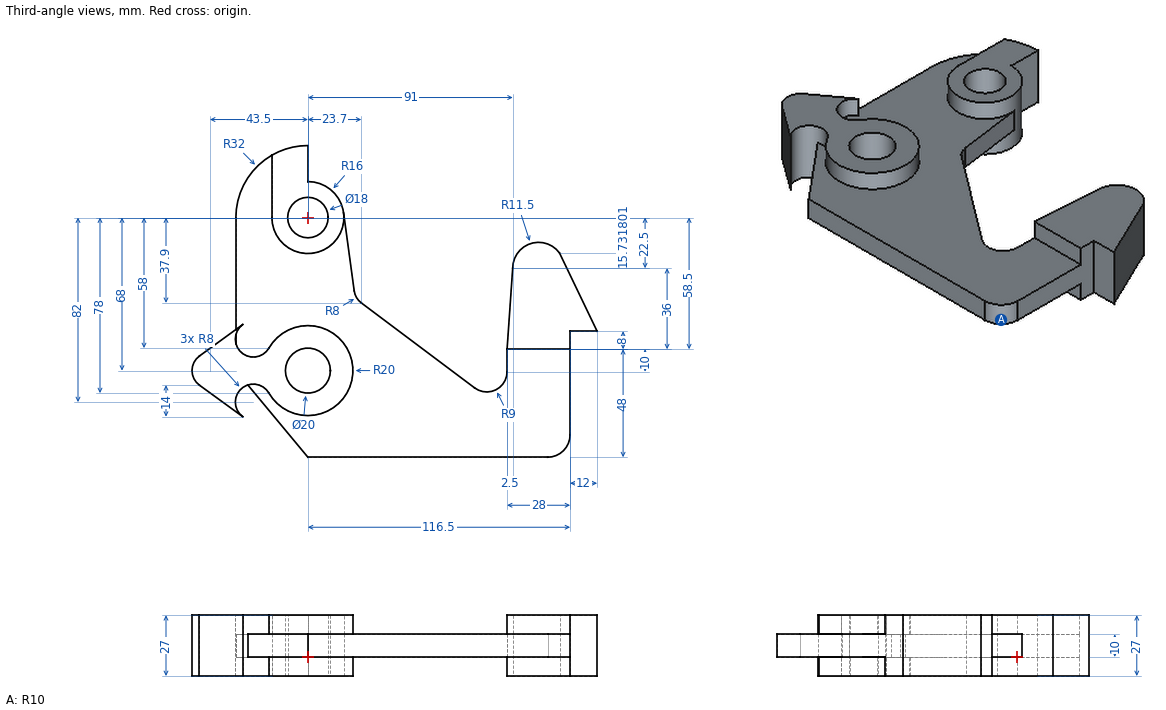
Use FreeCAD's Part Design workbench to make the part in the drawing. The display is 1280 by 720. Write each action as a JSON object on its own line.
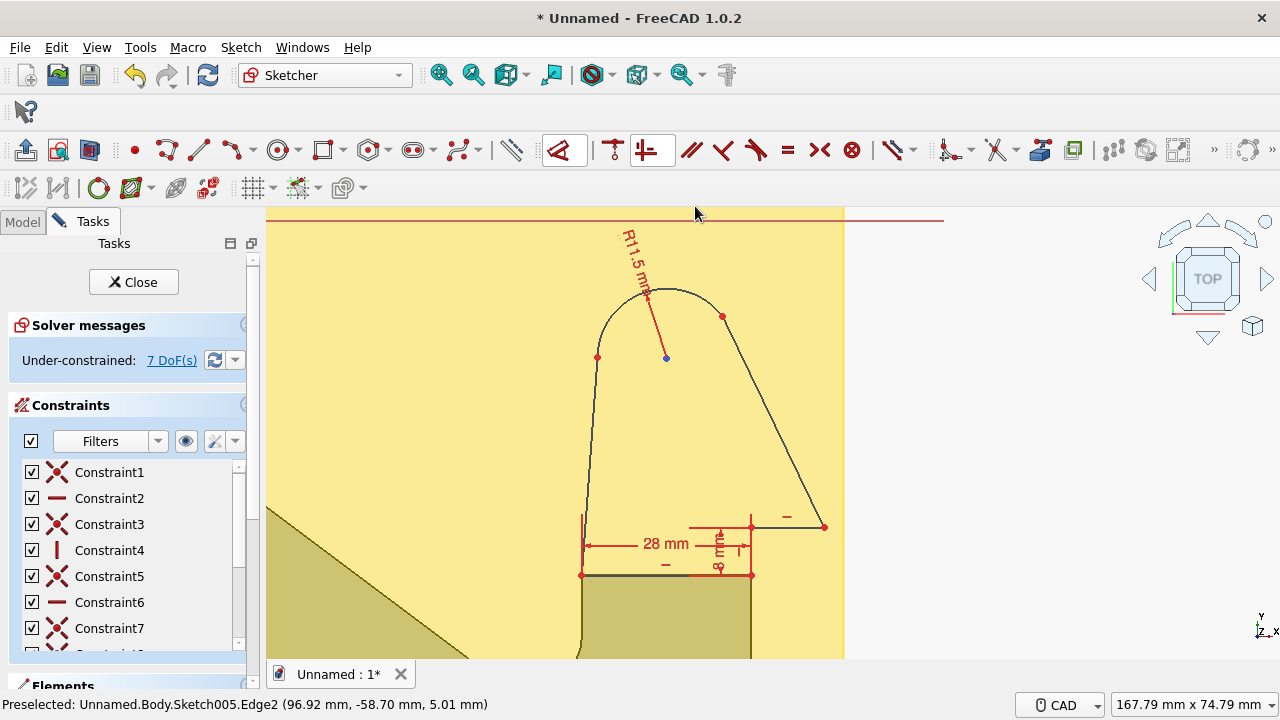
{"action": "left_click", "coordinate": [773, 528]}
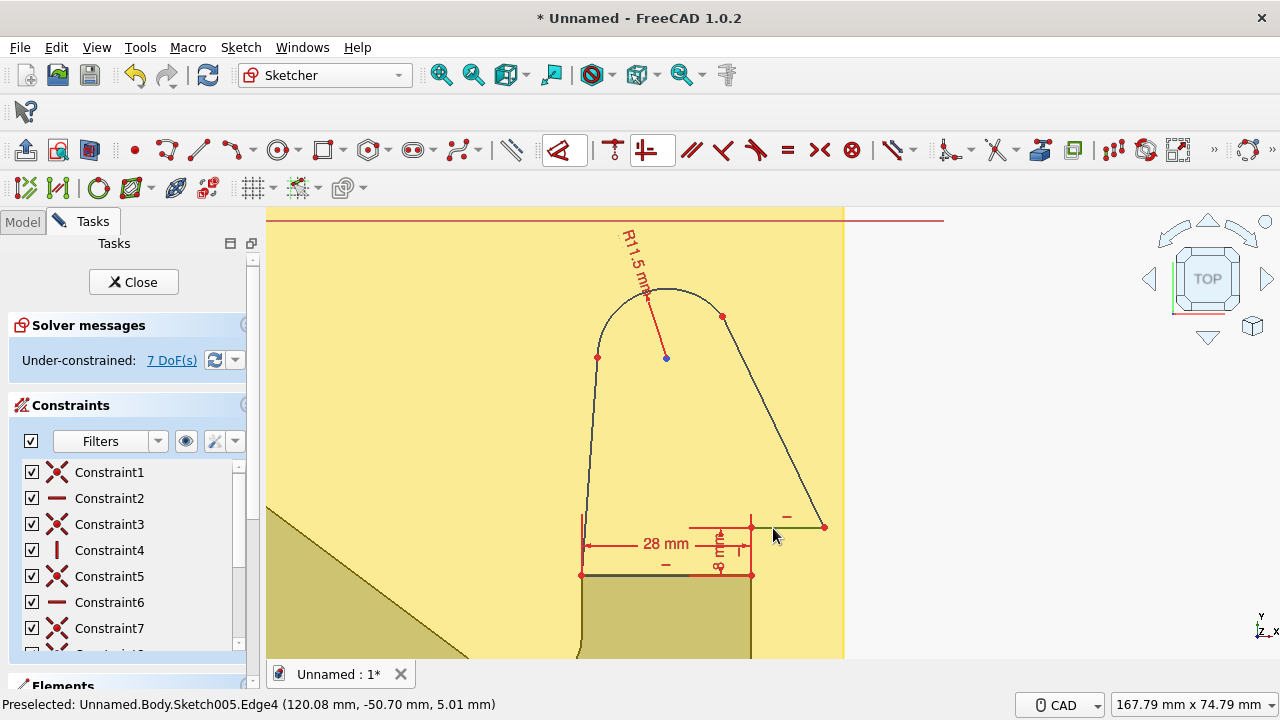
{"action": "left_click", "coordinate": [582, 150]}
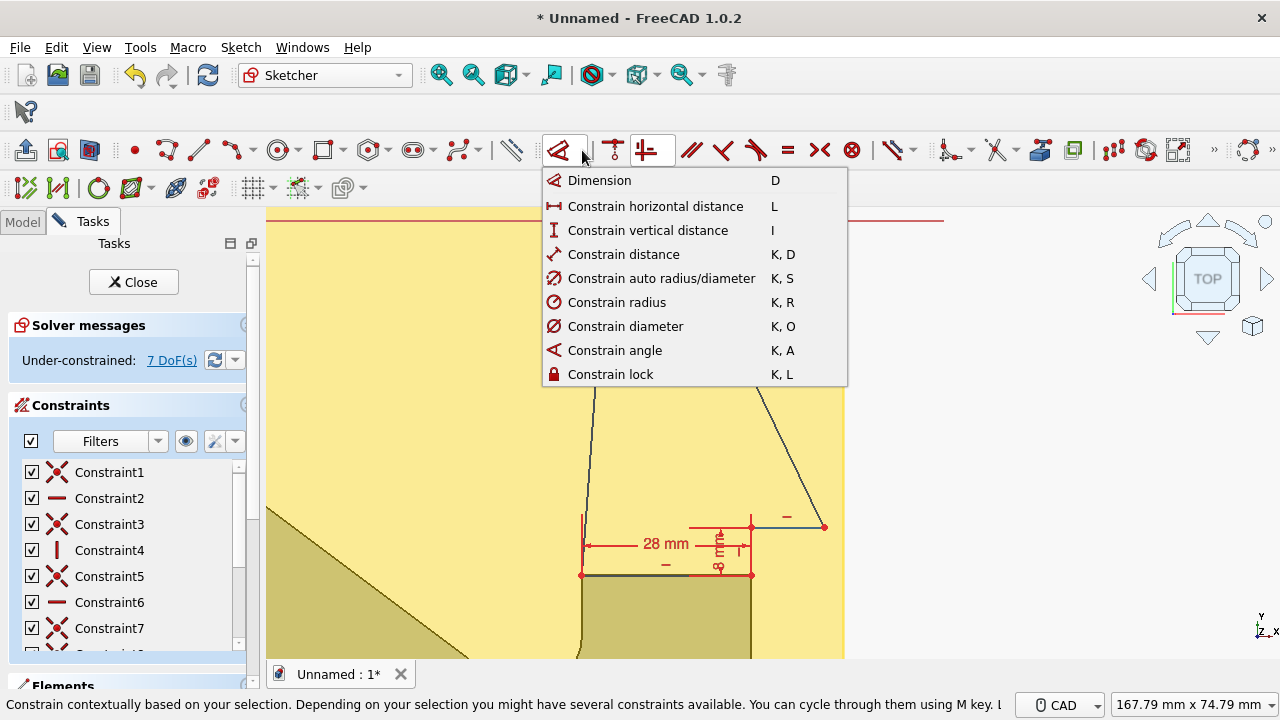
{"action": "left_click", "coordinate": [695, 206]}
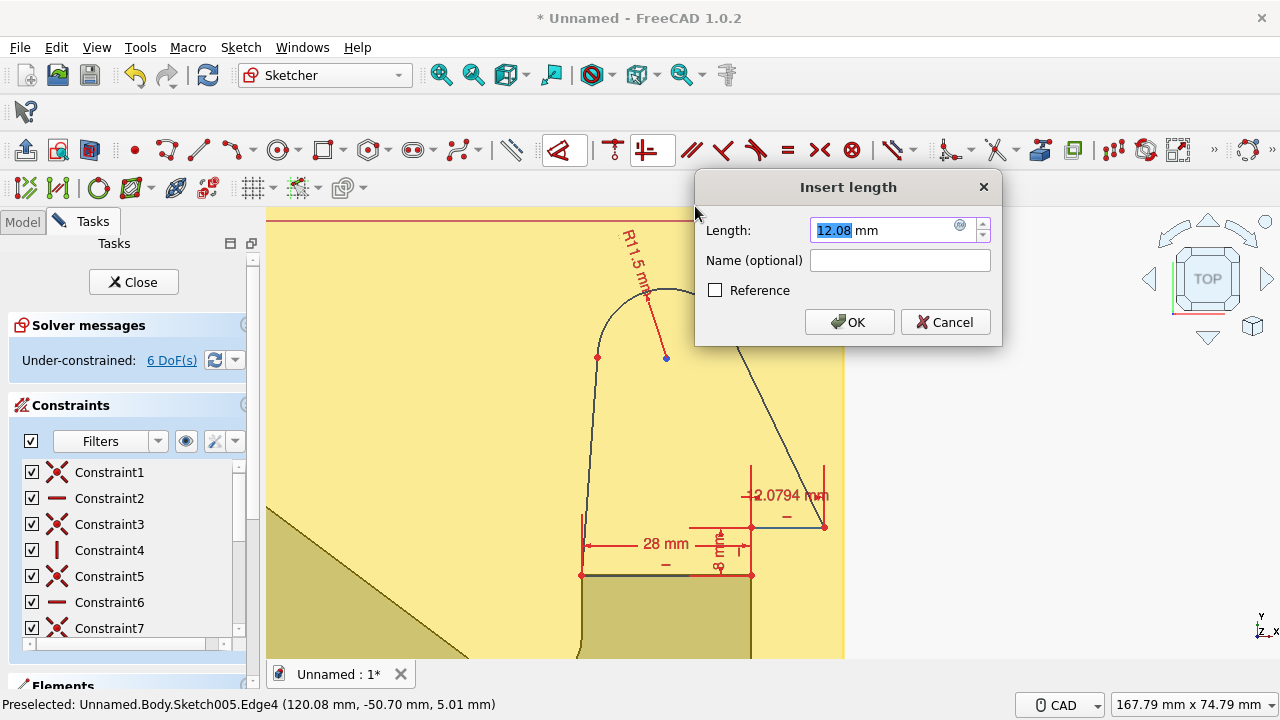
{"action": "type", "text": "12"}
{"action": "key", "text": "Return"}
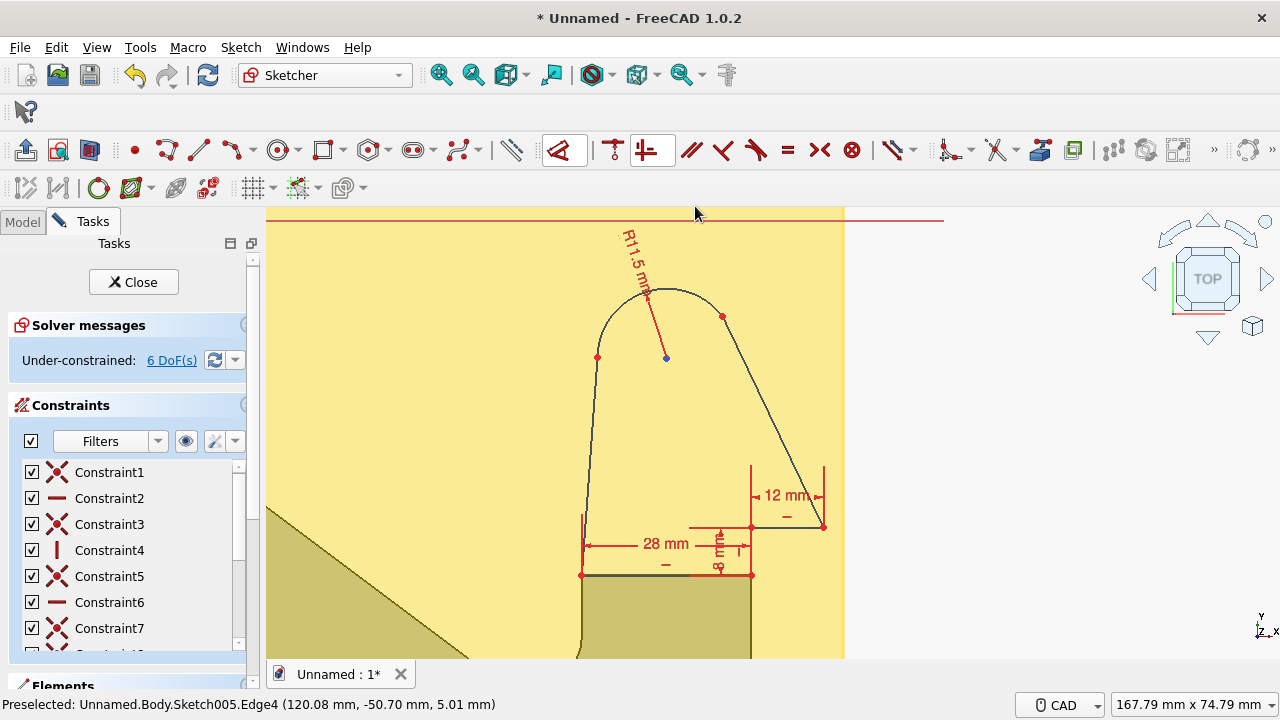
{"action": "left_click", "coordinate": [597, 358]}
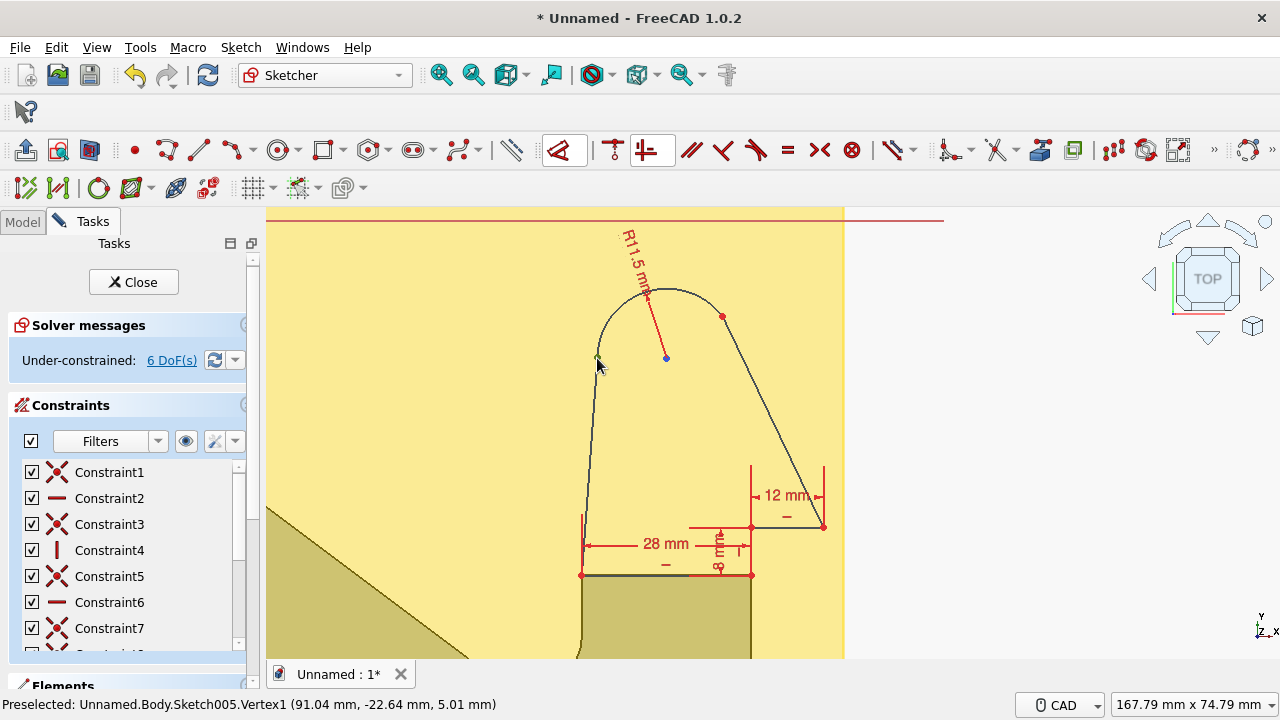
{"action": "left_click", "coordinate": [582, 150]}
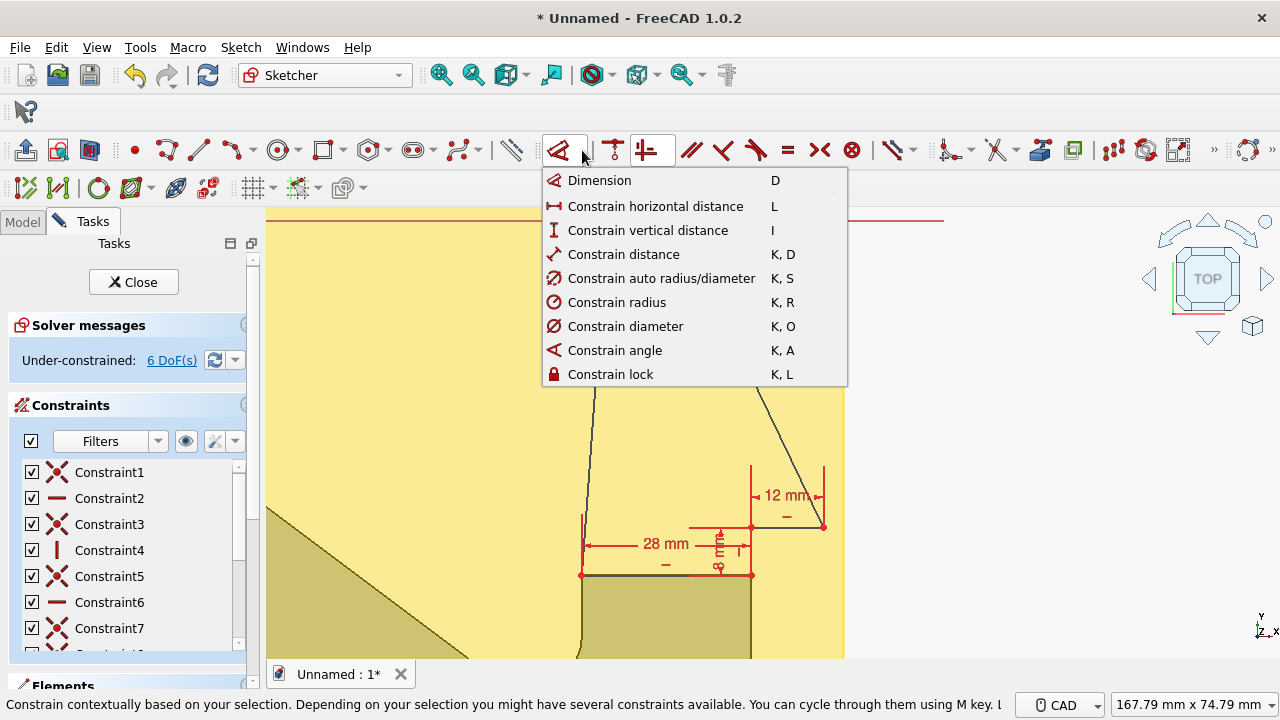
{"action": "left_click", "coordinate": [695, 206]}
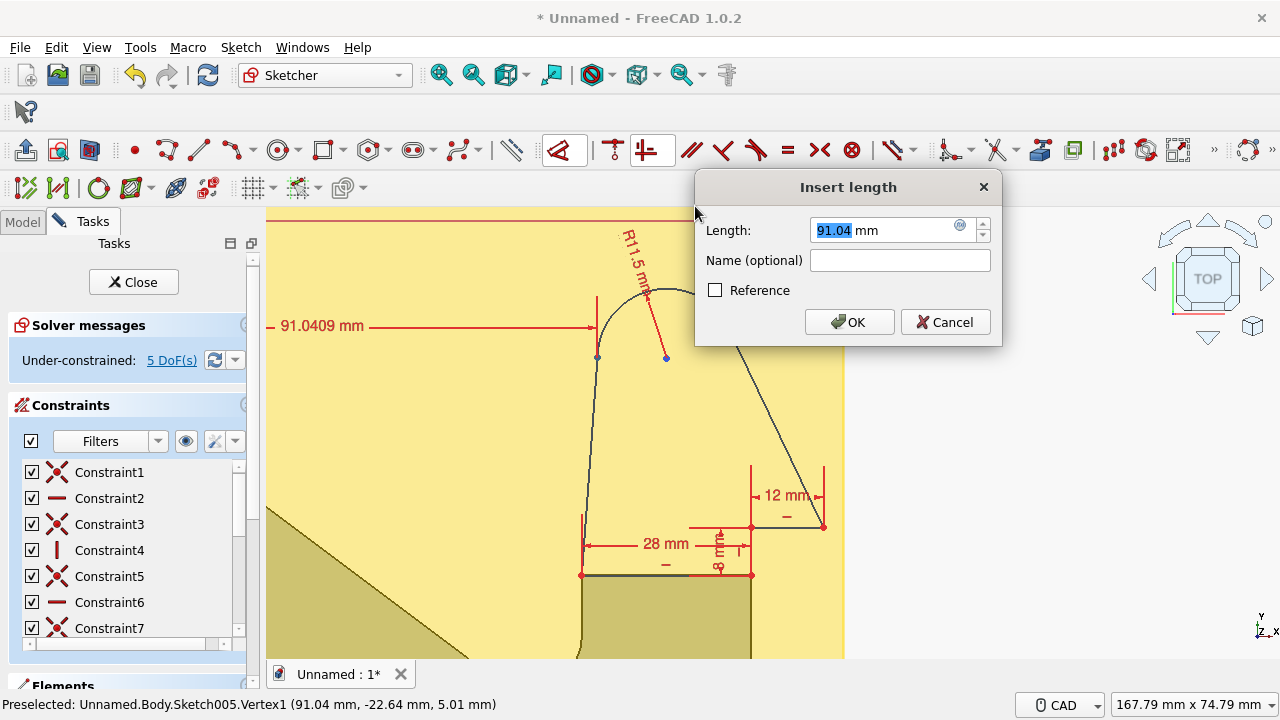
{"action": "type", "text": "91"}
{"action": "key", "text": "Return"}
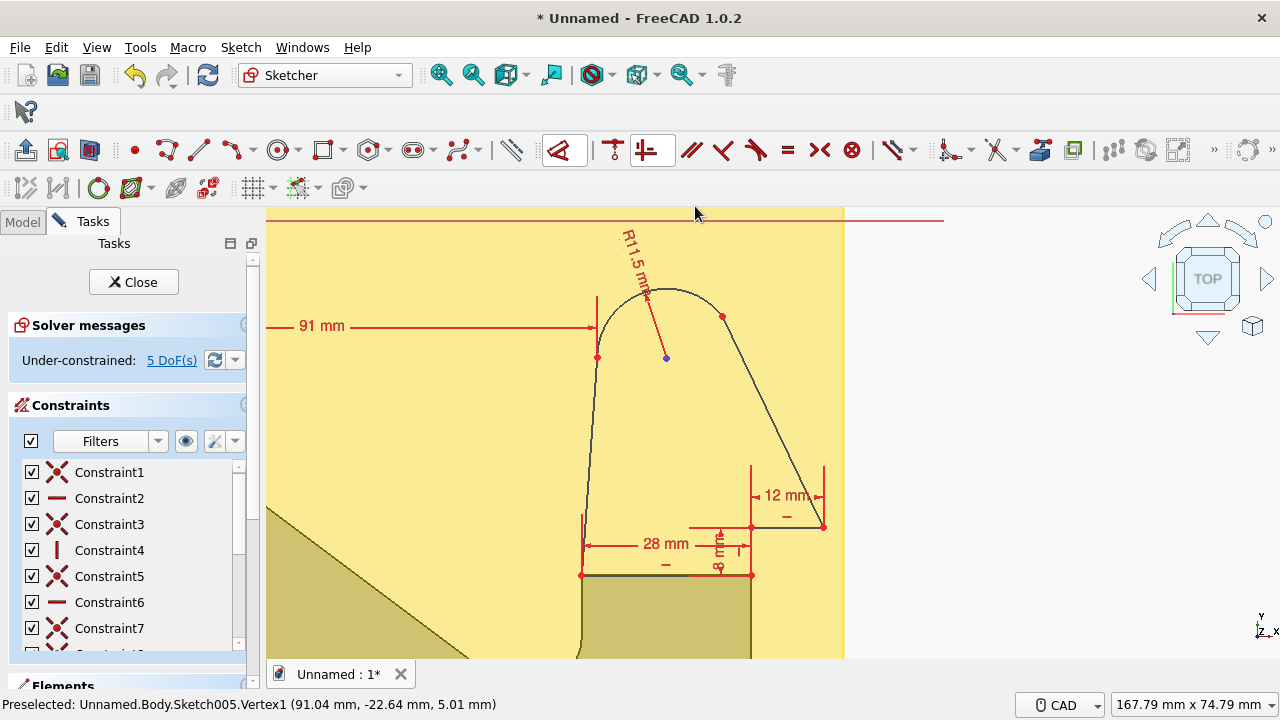
{"action": "left_click", "coordinate": [593, 423]}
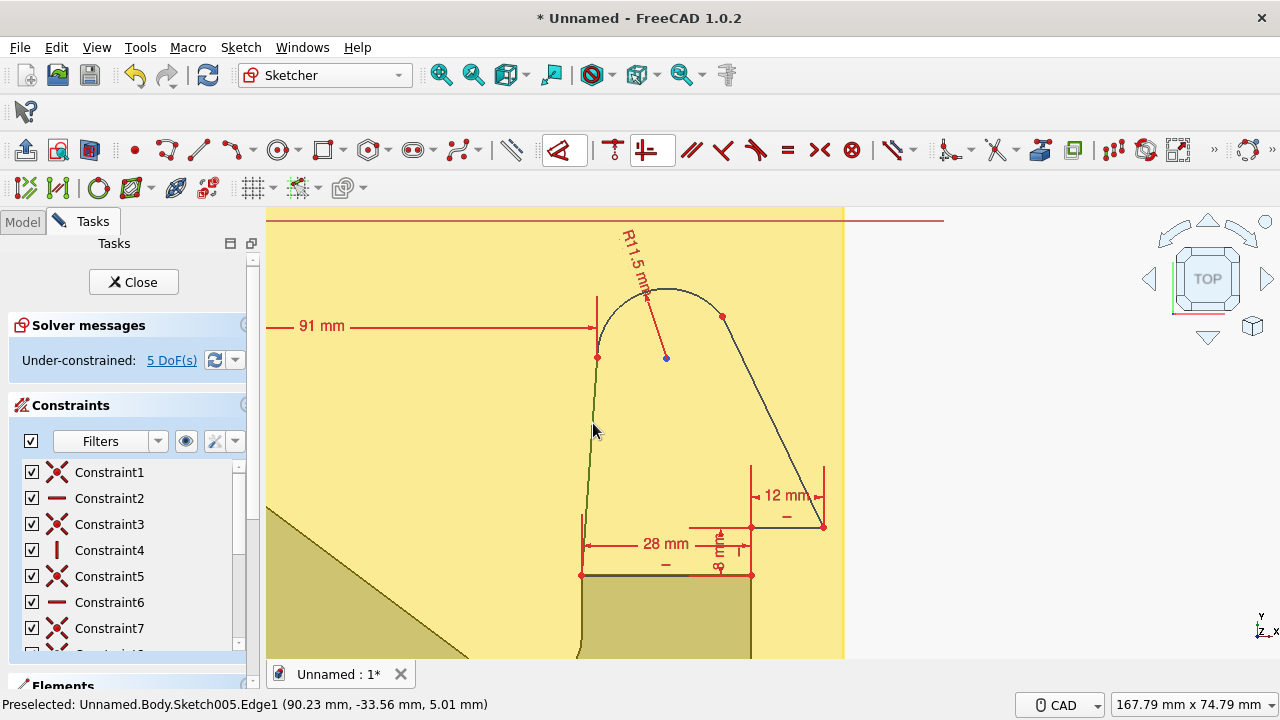
{"action": "left_click", "coordinate": [582, 150]}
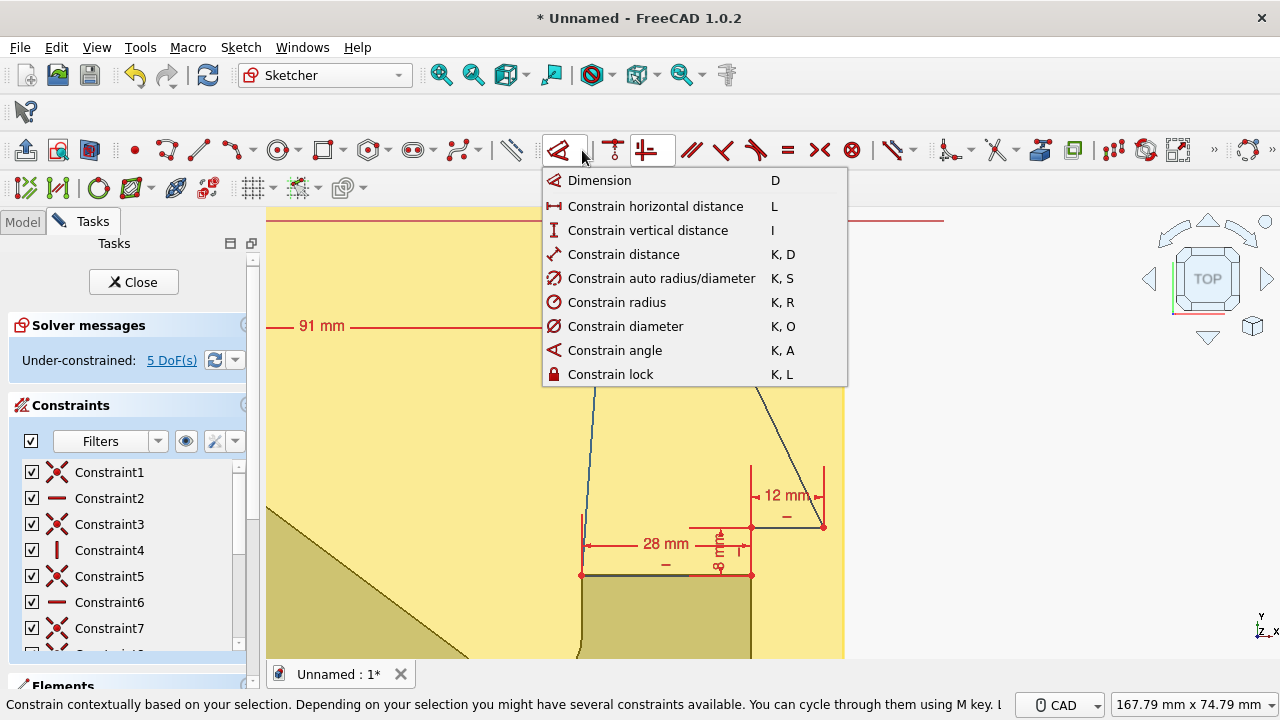
{"action": "left_click", "coordinate": [695, 230]}